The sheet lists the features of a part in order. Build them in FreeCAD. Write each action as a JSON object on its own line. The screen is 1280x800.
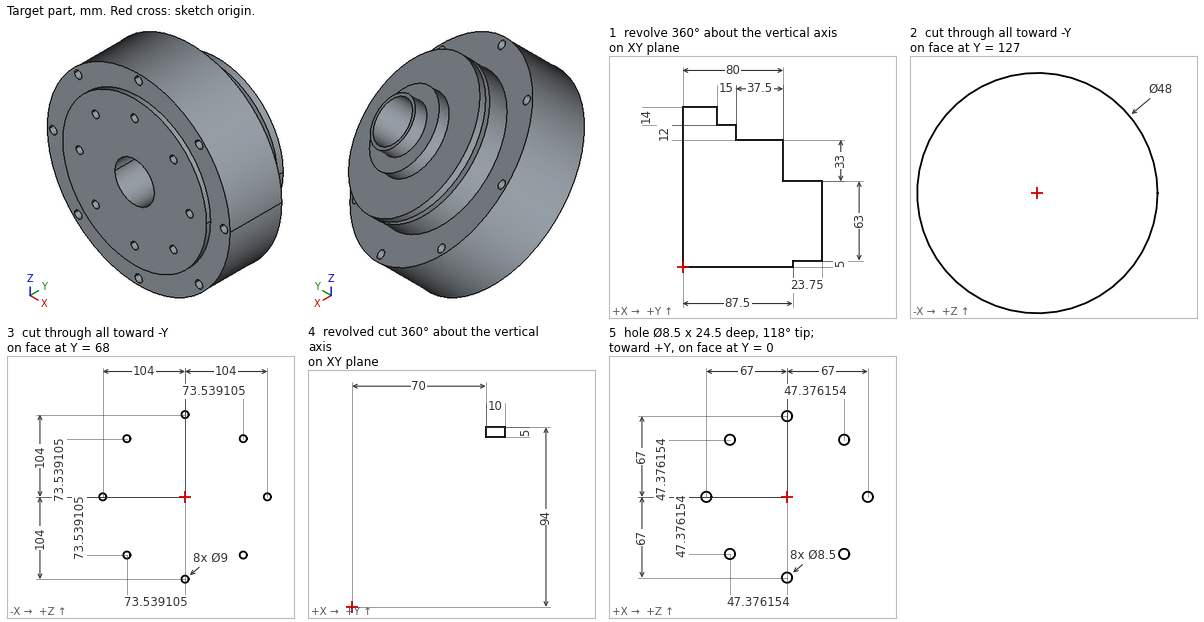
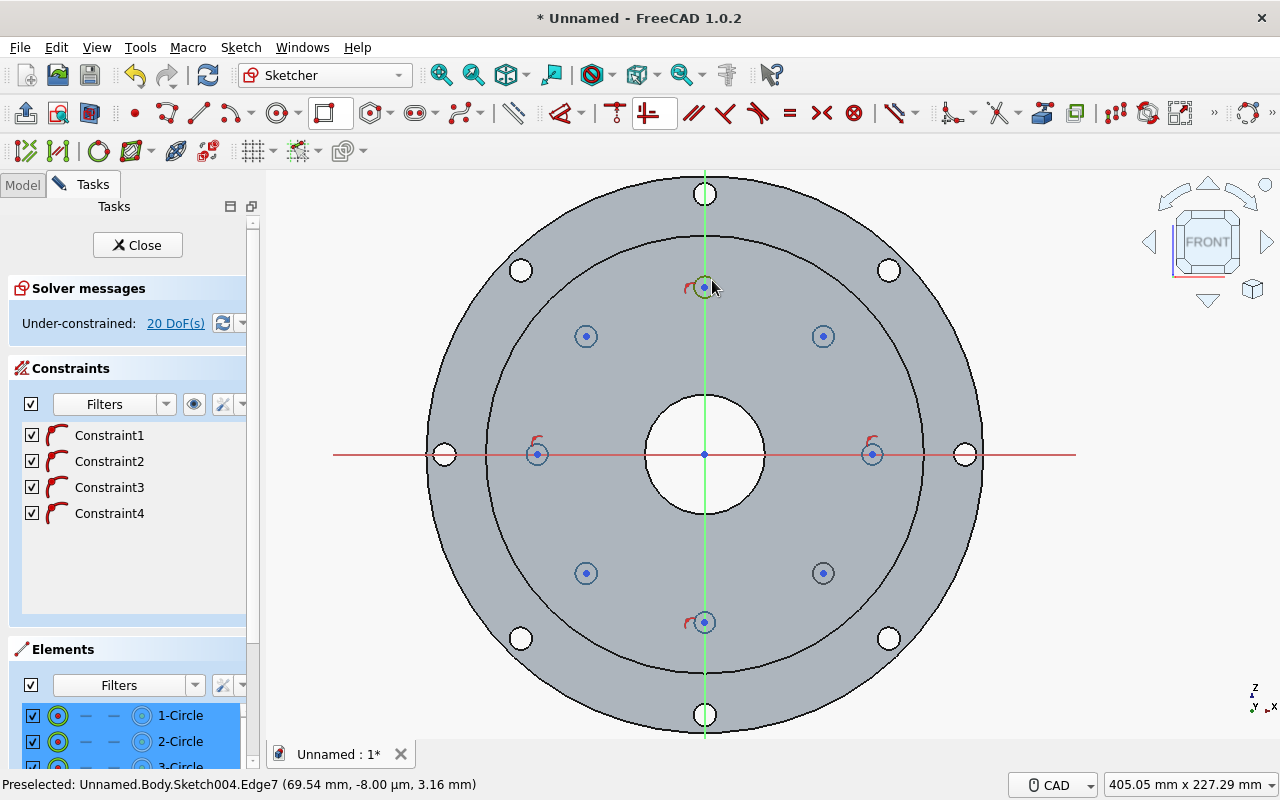
{"action": "scroll", "coordinate": [831, 566], "scroll_direction": "up", "scroll_amount": 2}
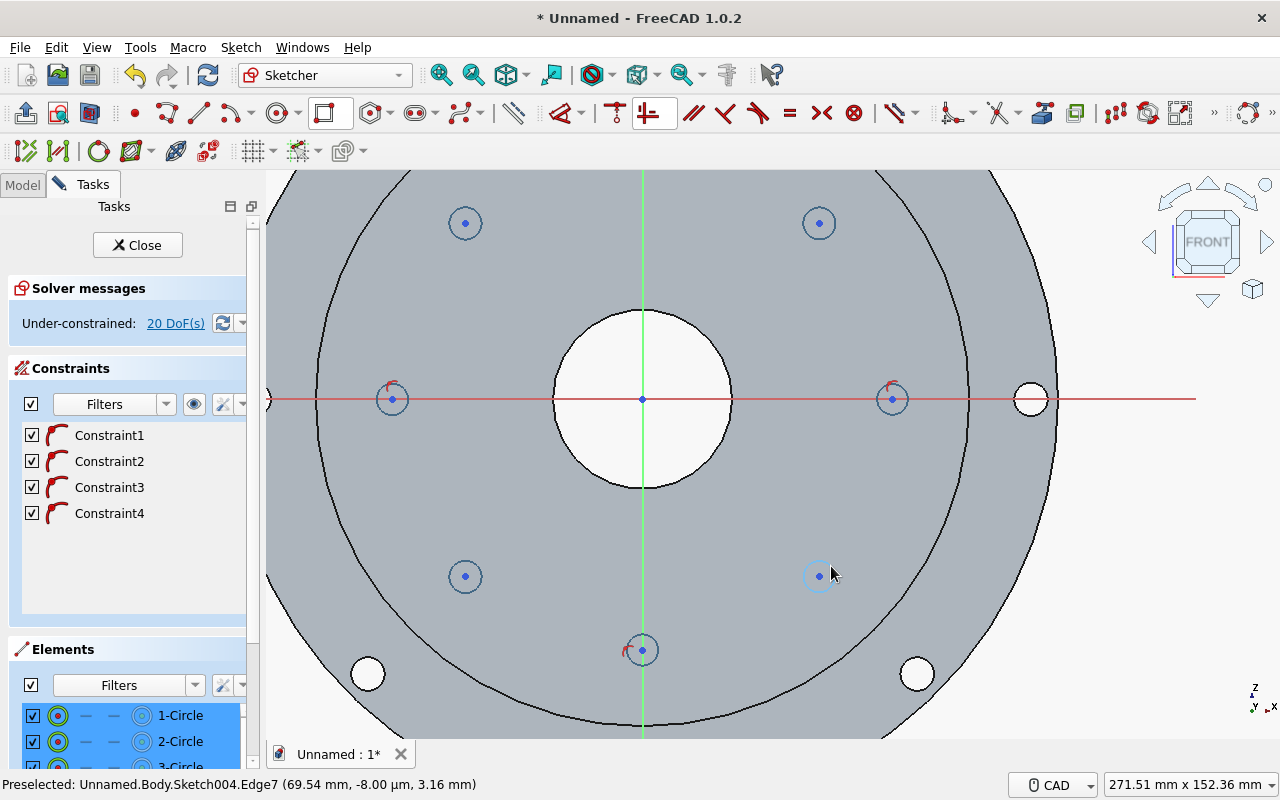
{"action": "left_click", "coordinate": [830, 566]}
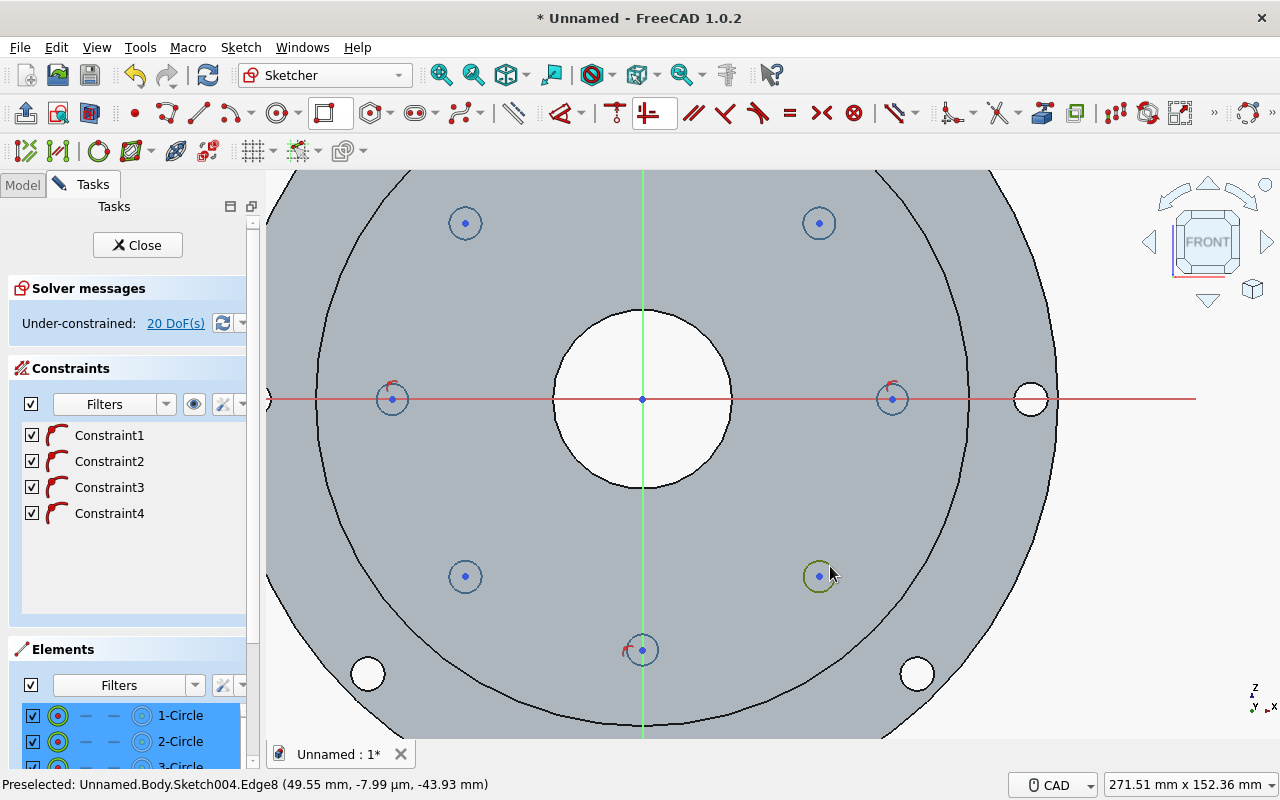
{"action": "left_click", "coordinate": [790, 114]}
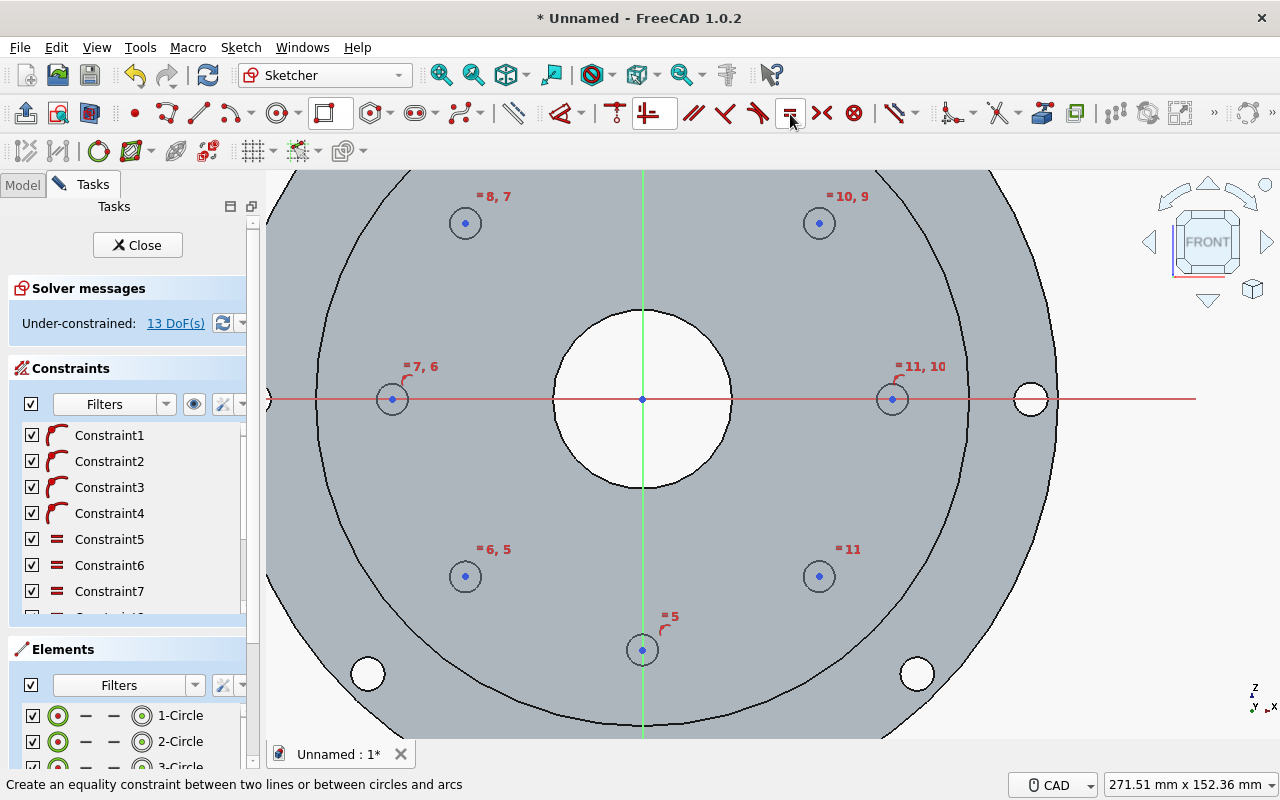
{"action": "left_click", "coordinate": [465, 577]}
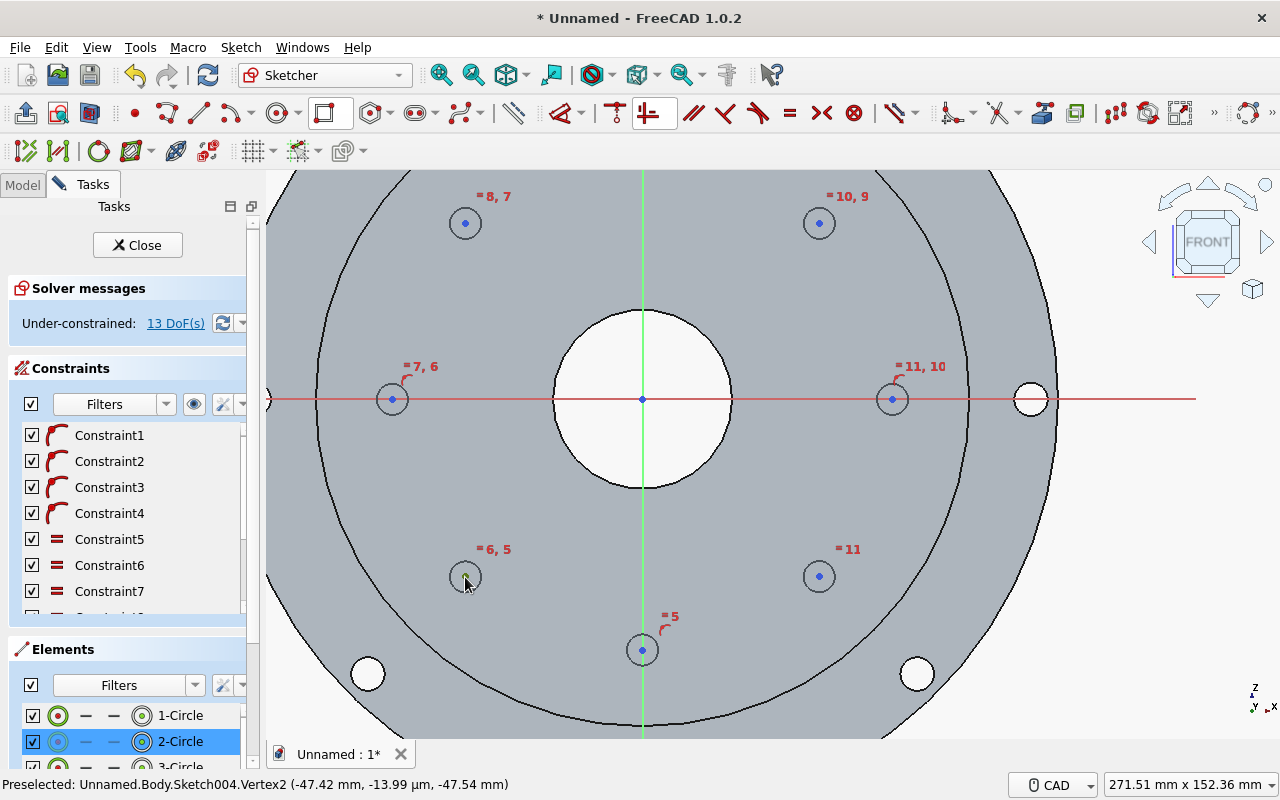
{"action": "left_click", "coordinate": [465, 223]}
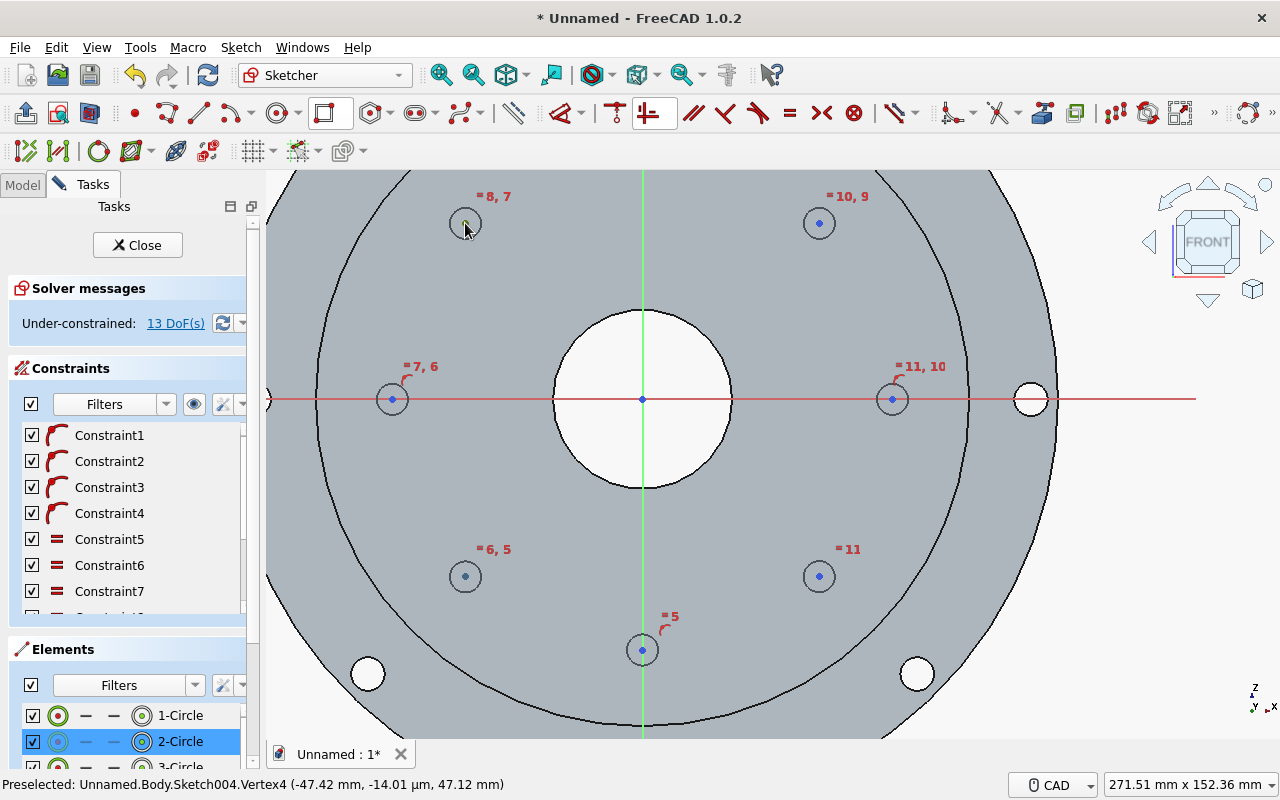
{"action": "key", "text": "v"}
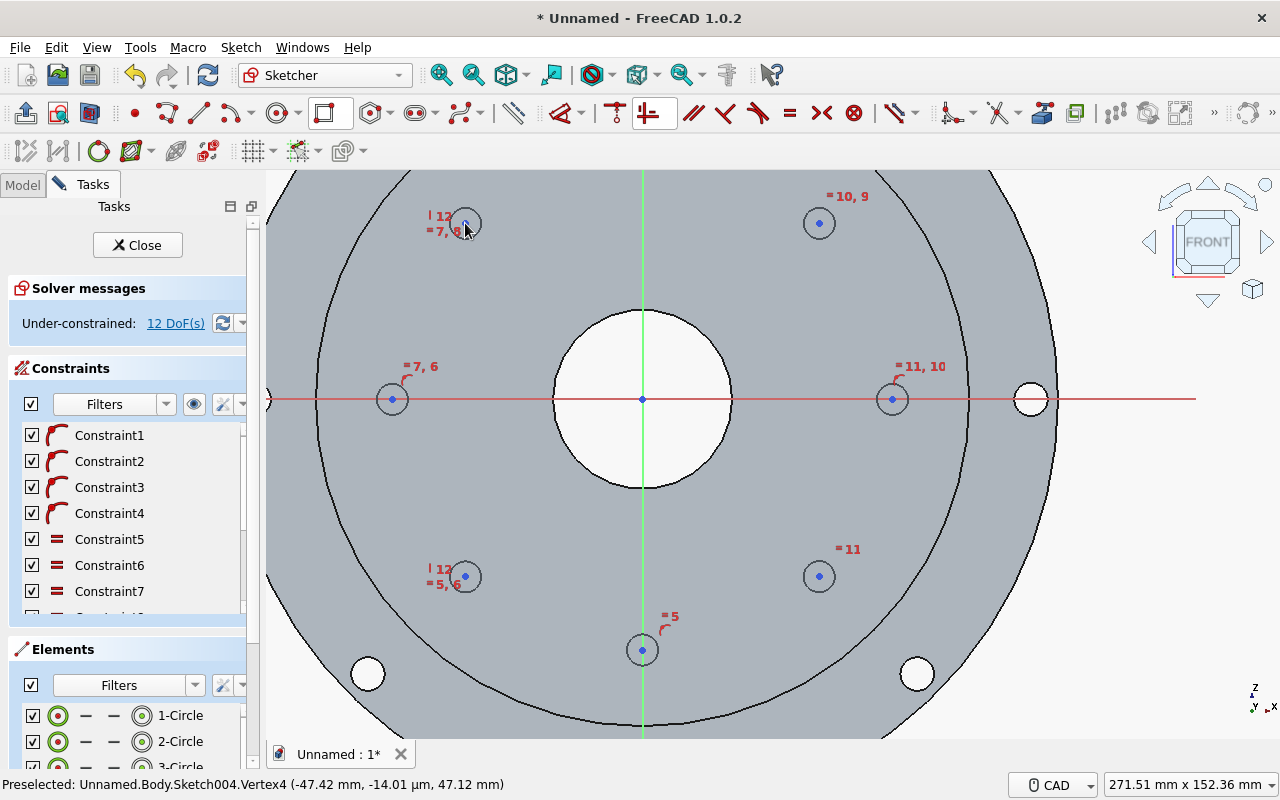
{"action": "left_click", "coordinate": [465, 223]}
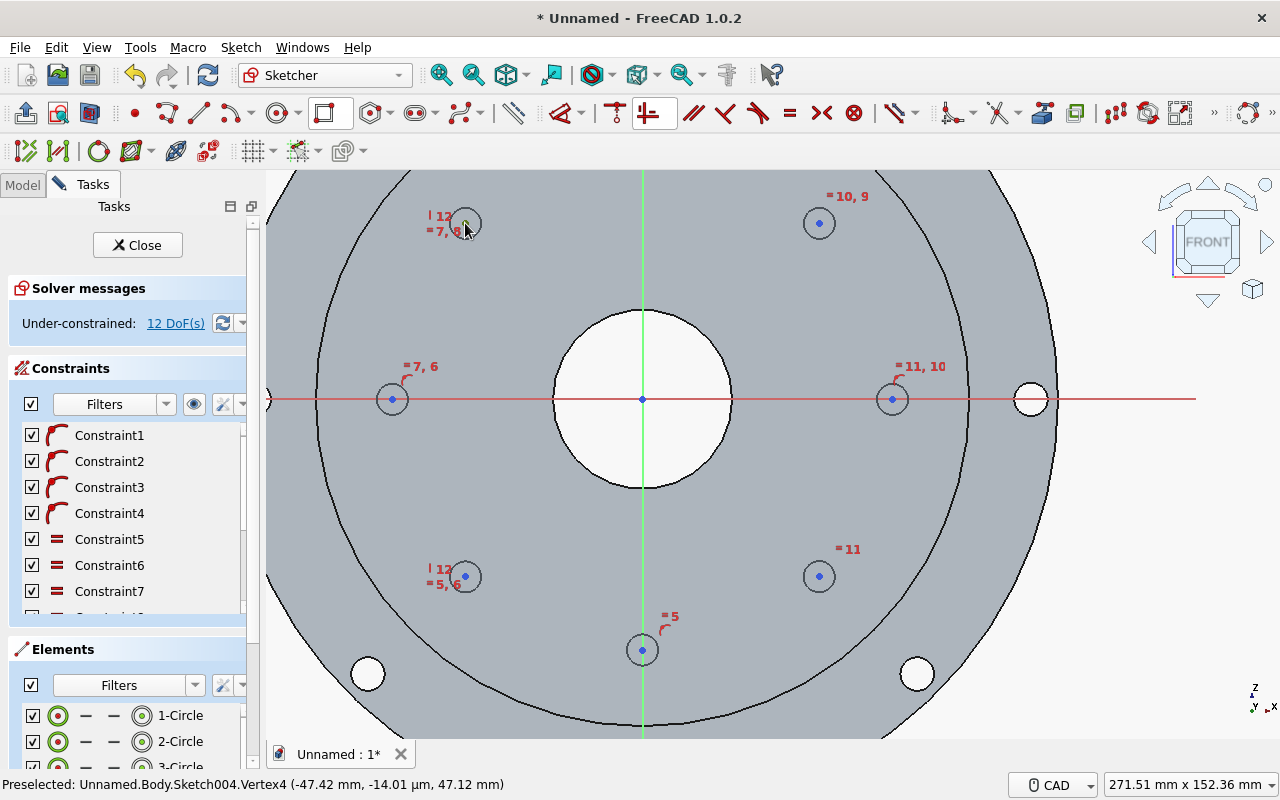
{"action": "left_click", "coordinate": [819, 223]}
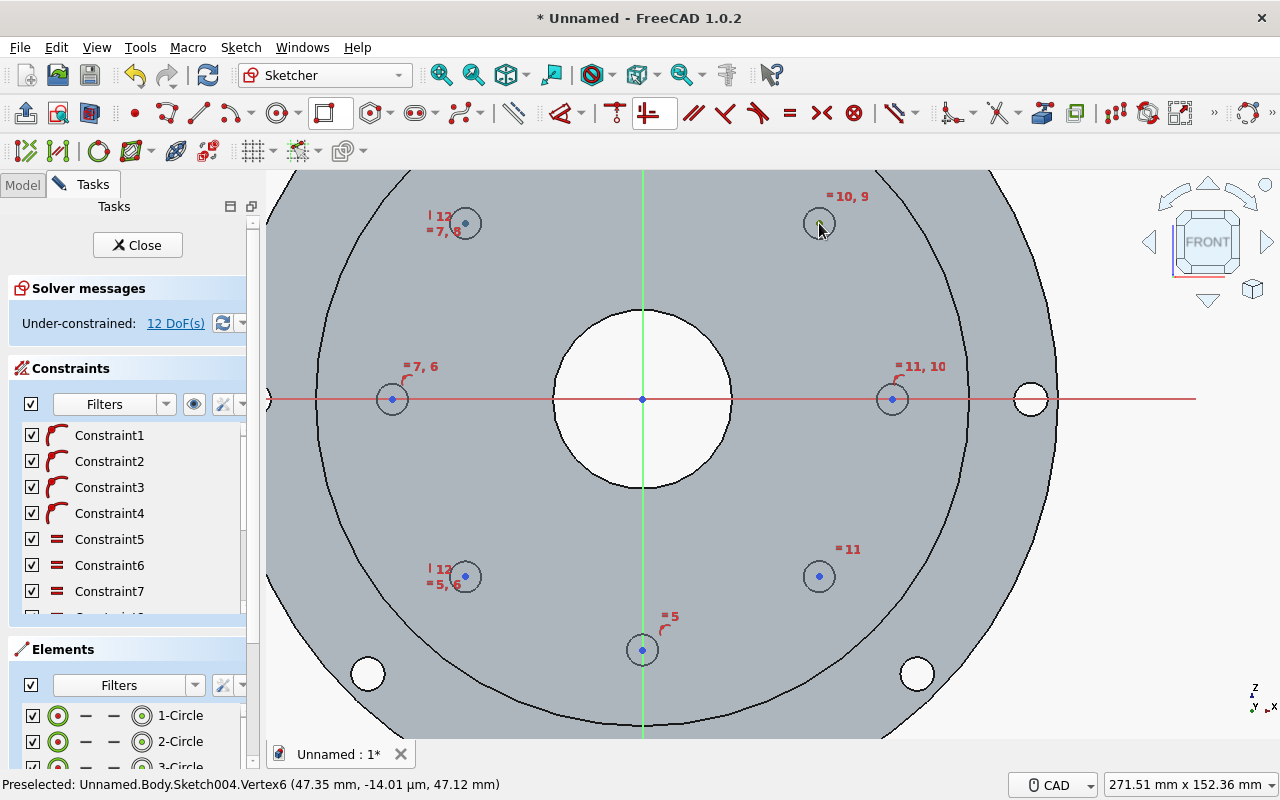
{"action": "left_click", "coordinate": [672, 114]}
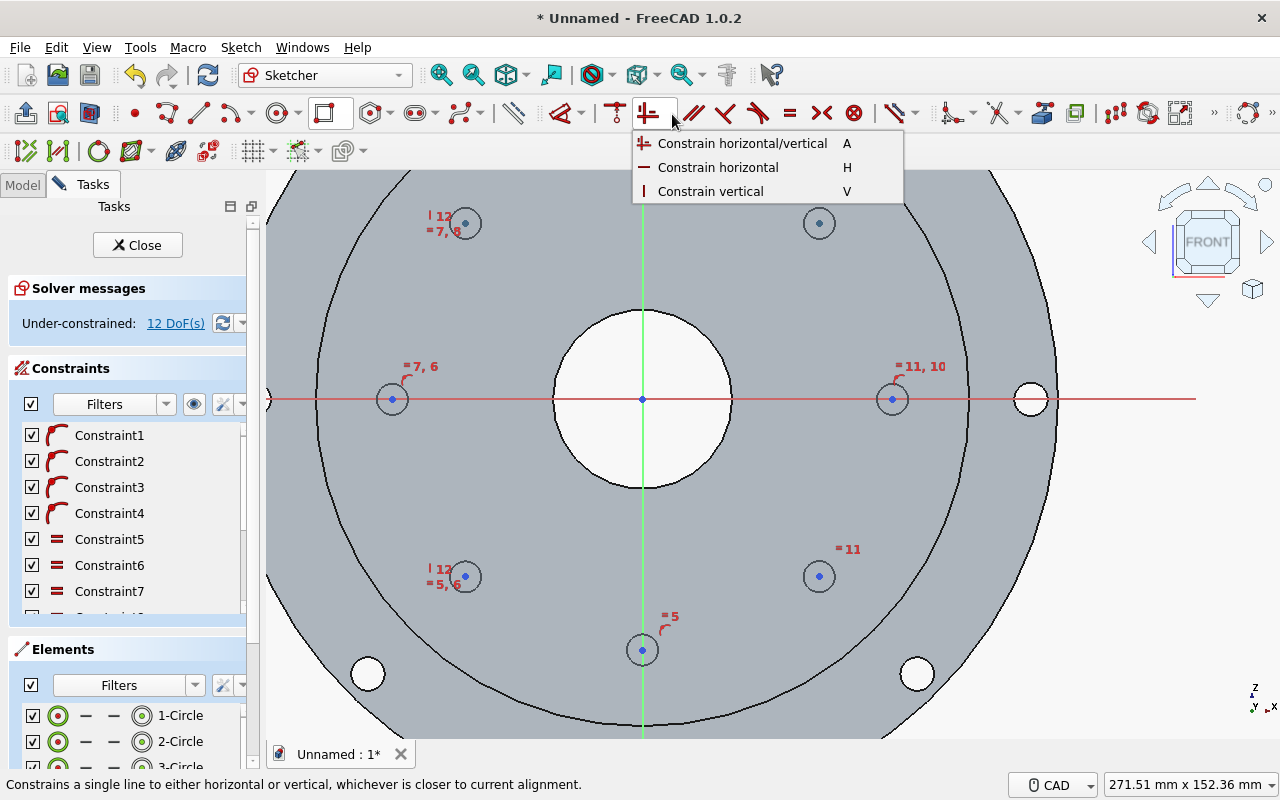
{"action": "left_click", "coordinate": [768, 167]}